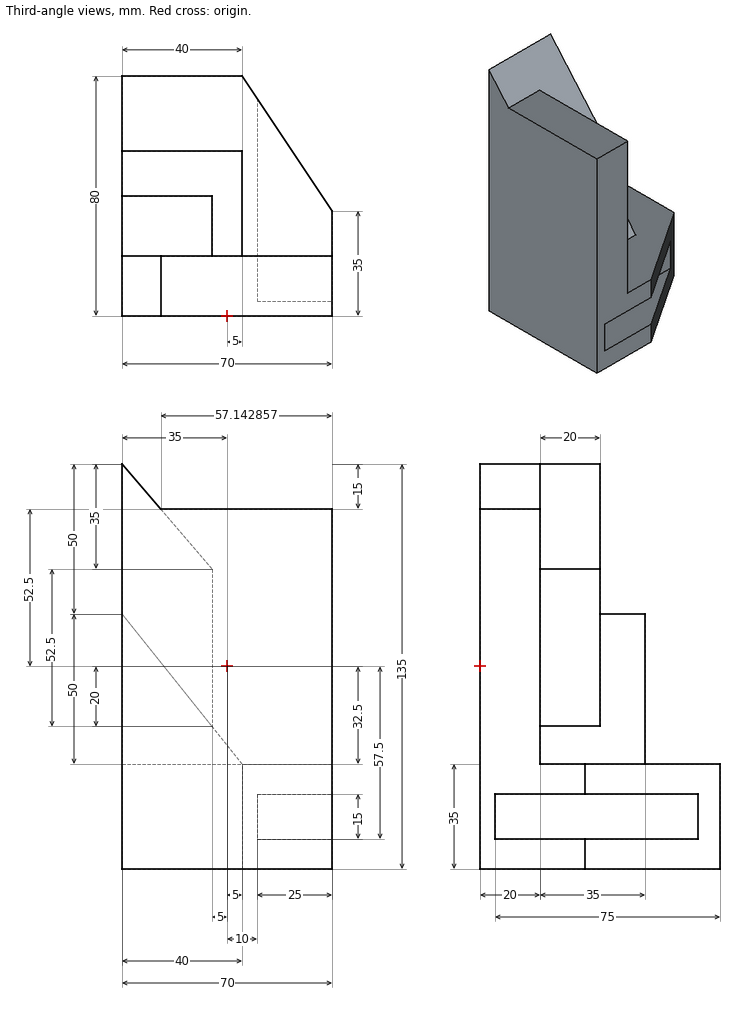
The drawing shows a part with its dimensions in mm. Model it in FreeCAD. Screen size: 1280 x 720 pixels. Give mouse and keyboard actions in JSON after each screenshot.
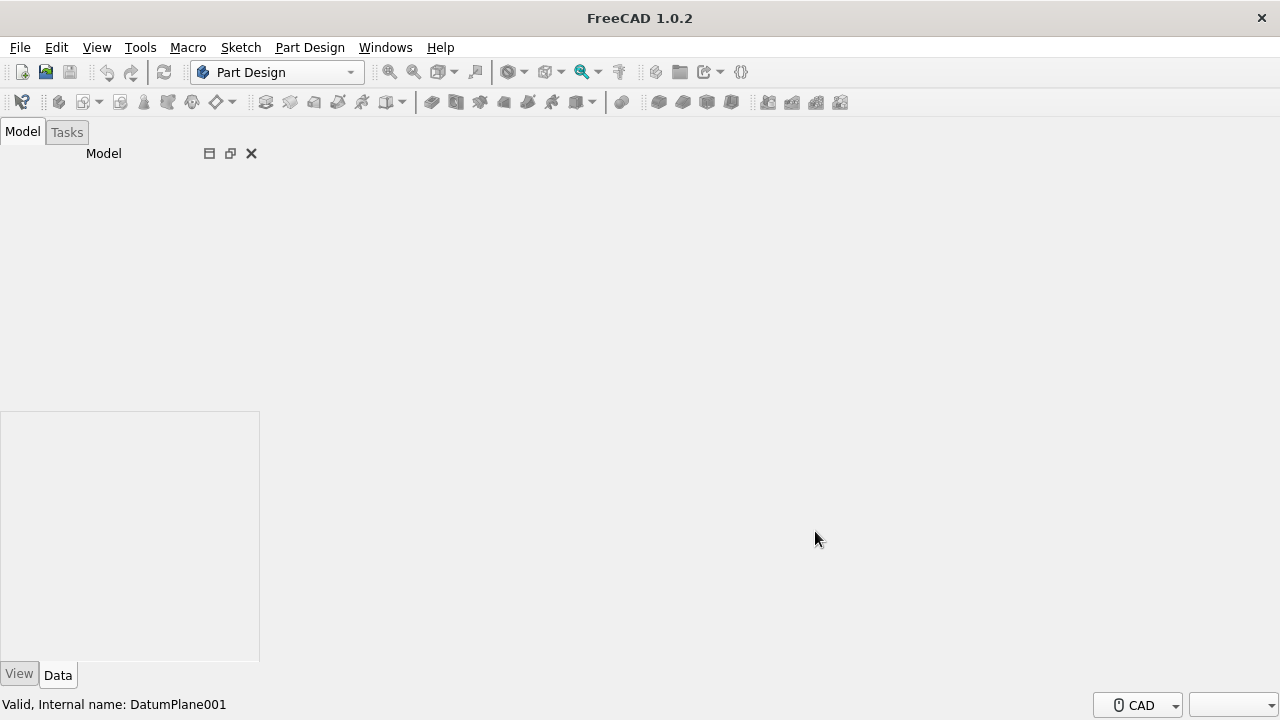
{"action": "left_click", "coordinate": [22, 72]}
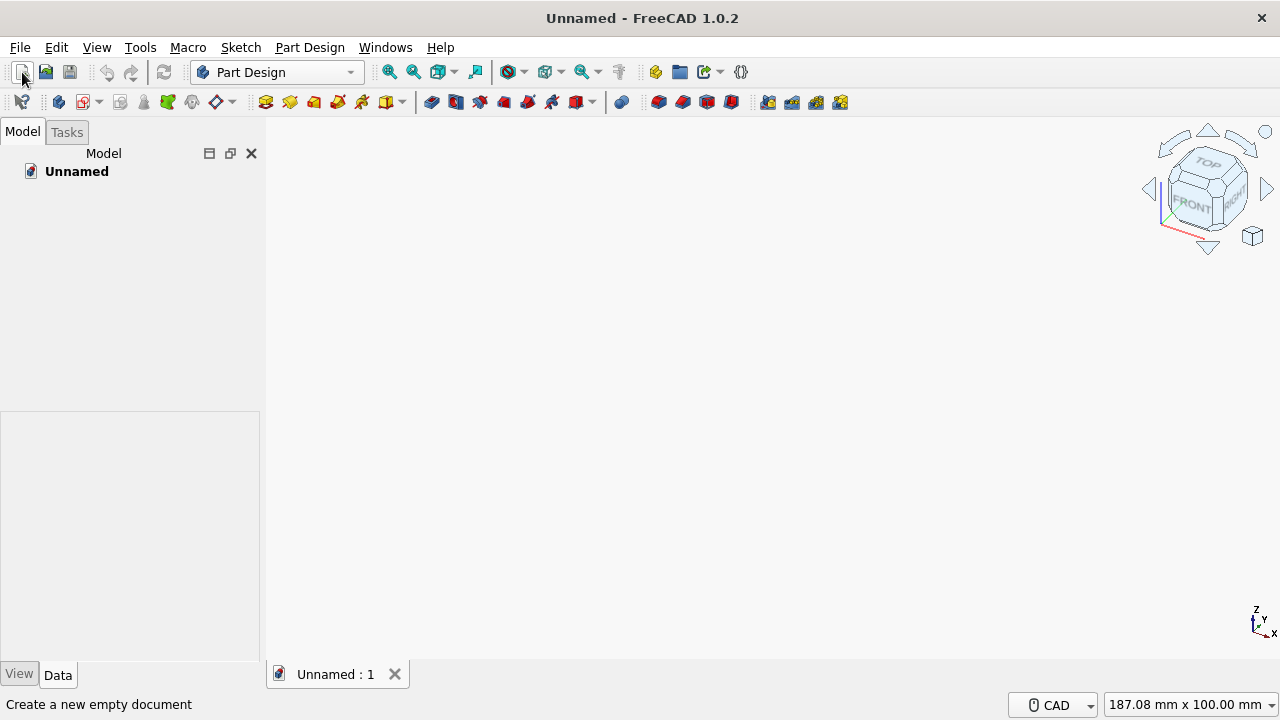
{"action": "left_click", "coordinate": [84, 102]}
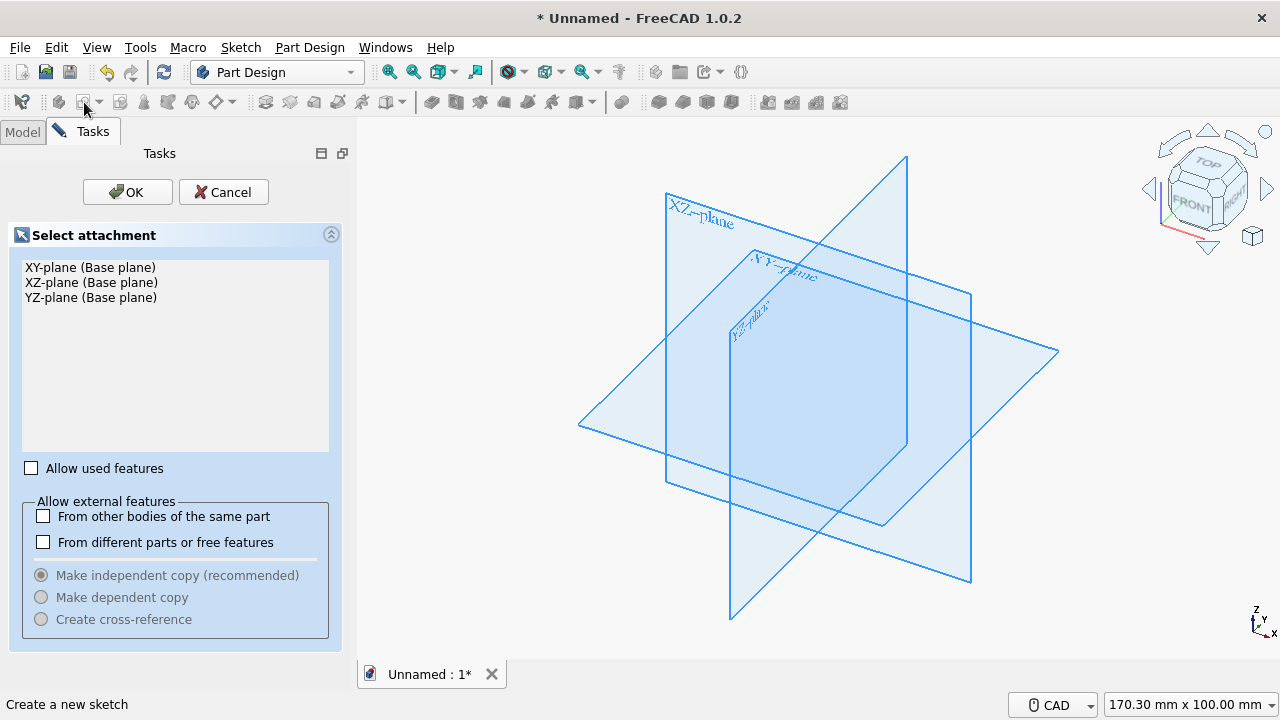
{"action": "left_click", "coordinate": [82, 282]}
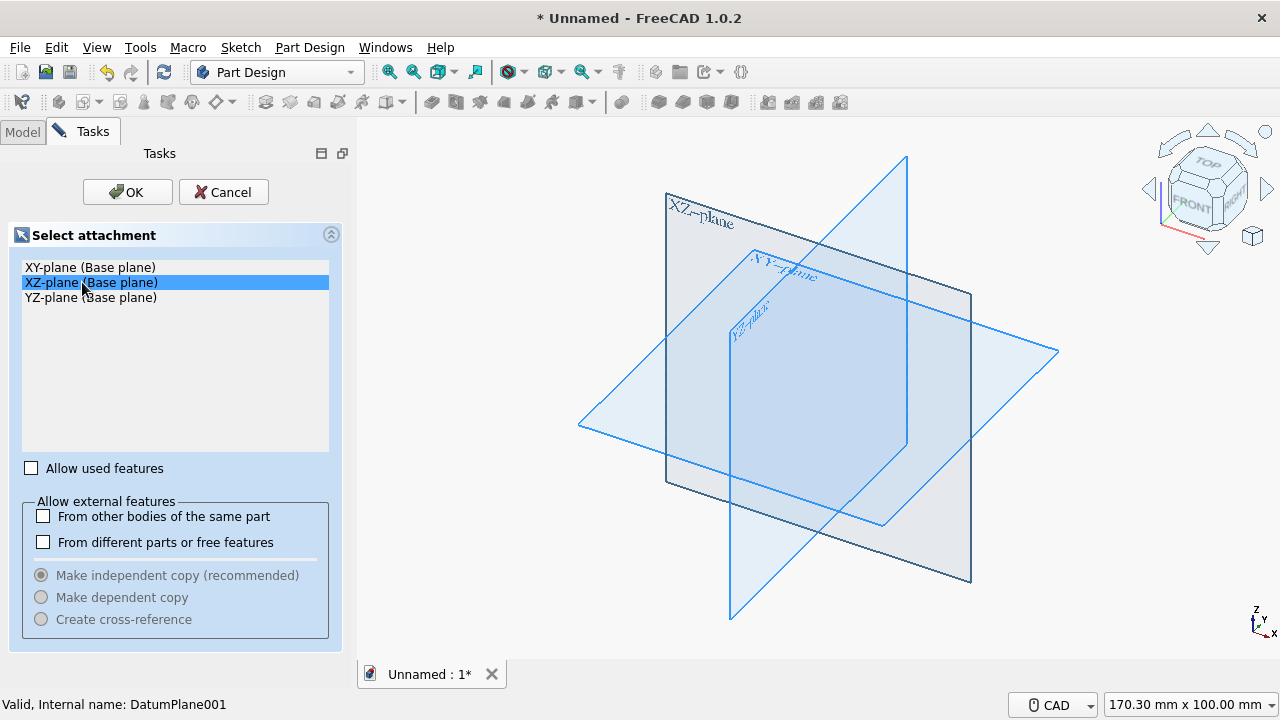
{"action": "left_click", "coordinate": [128, 192]}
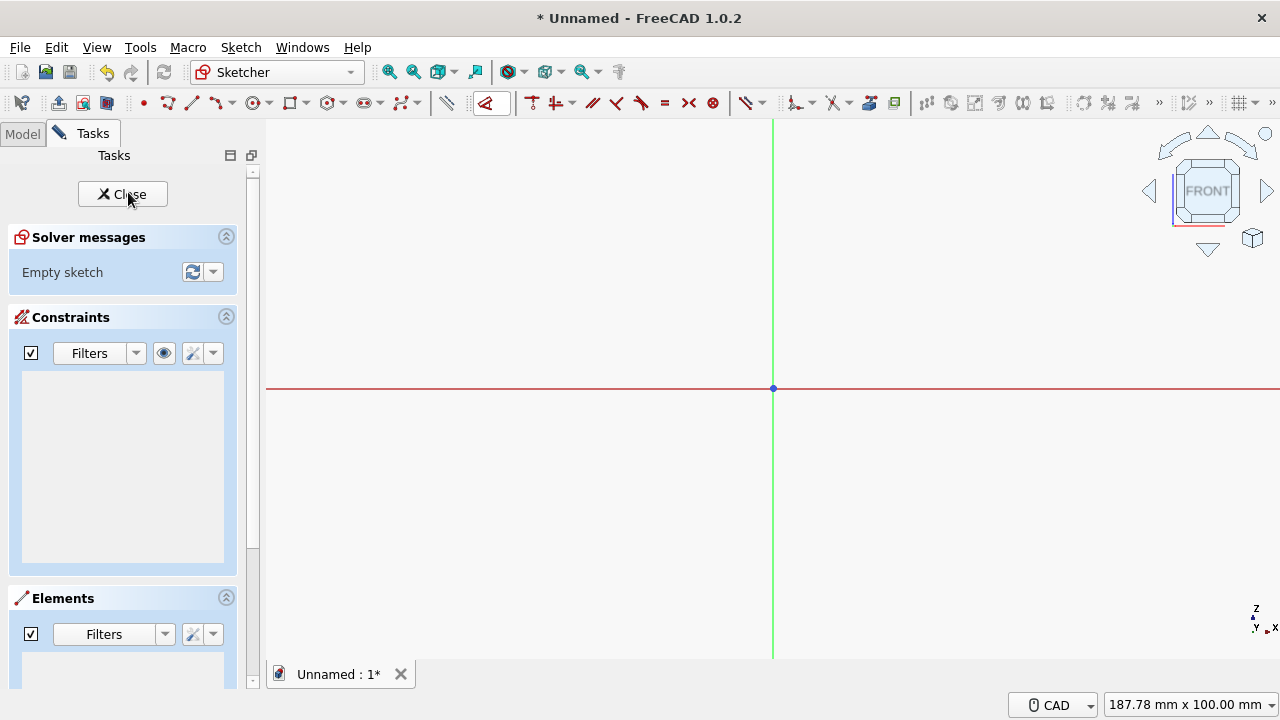
{"action": "scroll", "coordinate": [649, 389], "scroll_direction": "down", "scroll_amount": 4}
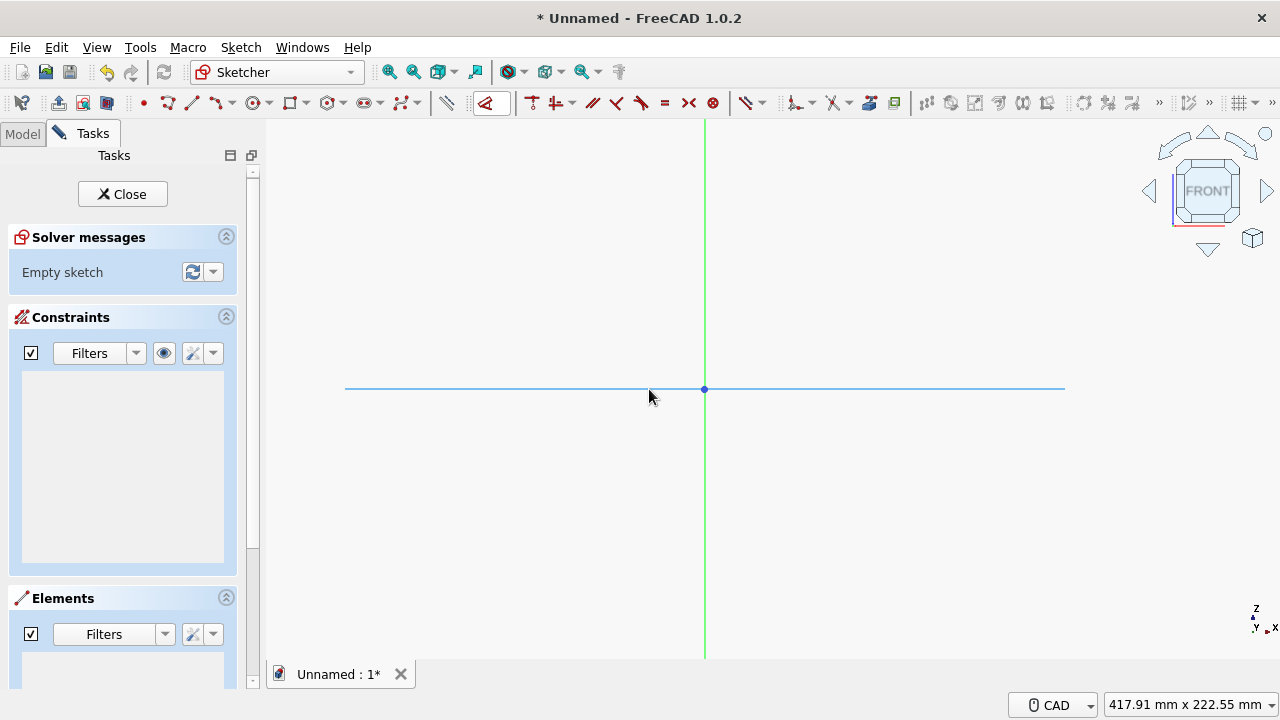
{"action": "key", "text": "g v"}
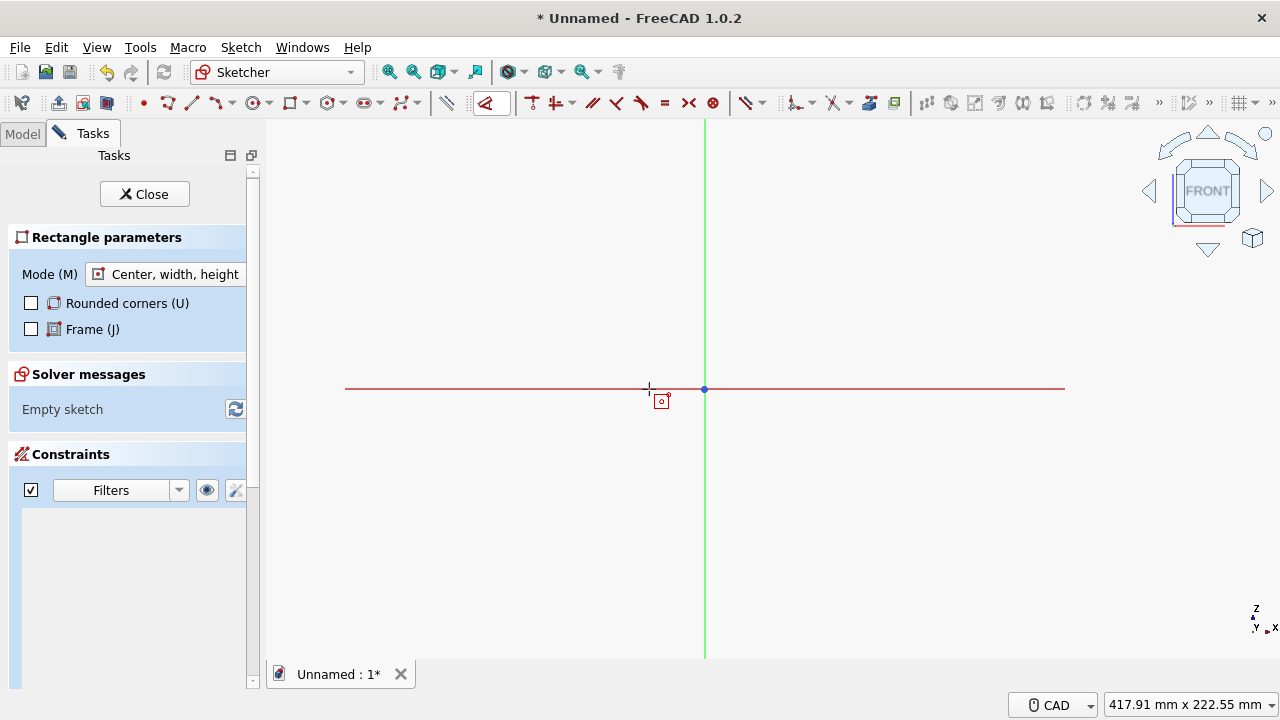
{"action": "left_click", "coordinate": [705, 389]}
{"action": "left_click", "coordinate": [790, 225]}
{"action": "key", "text": "Escape"}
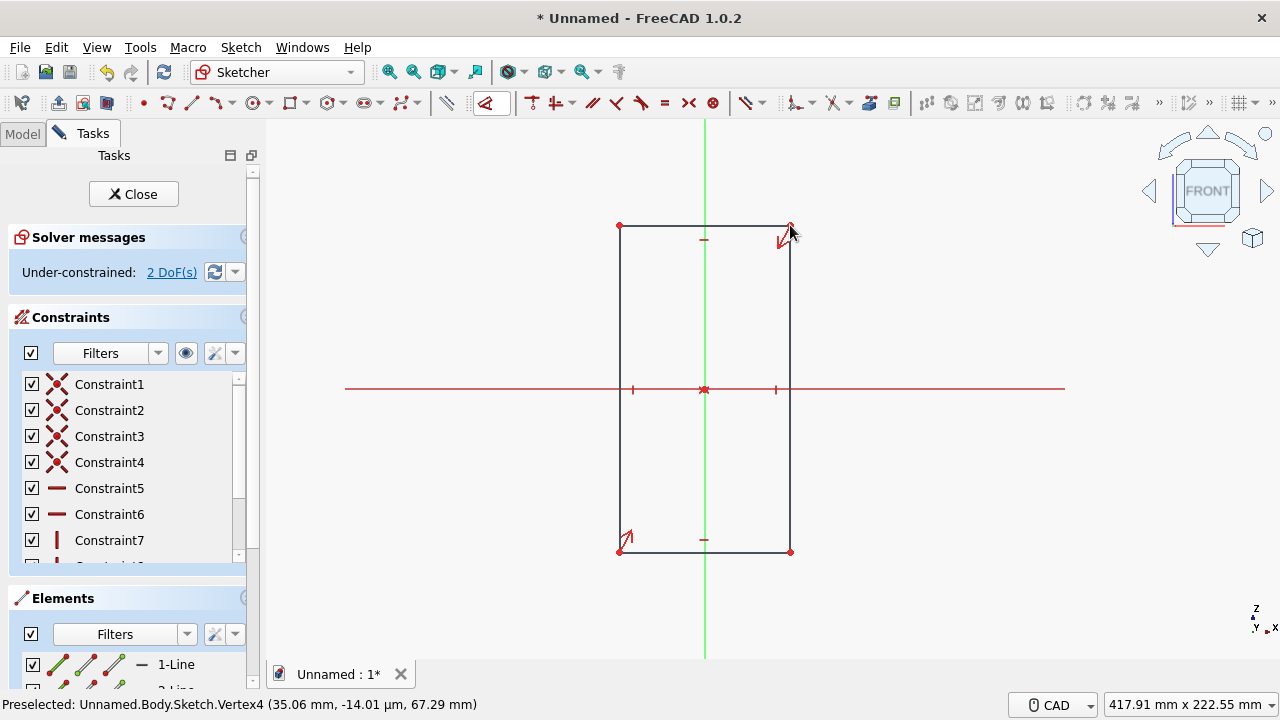
{"action": "left_click", "coordinate": [671, 553]}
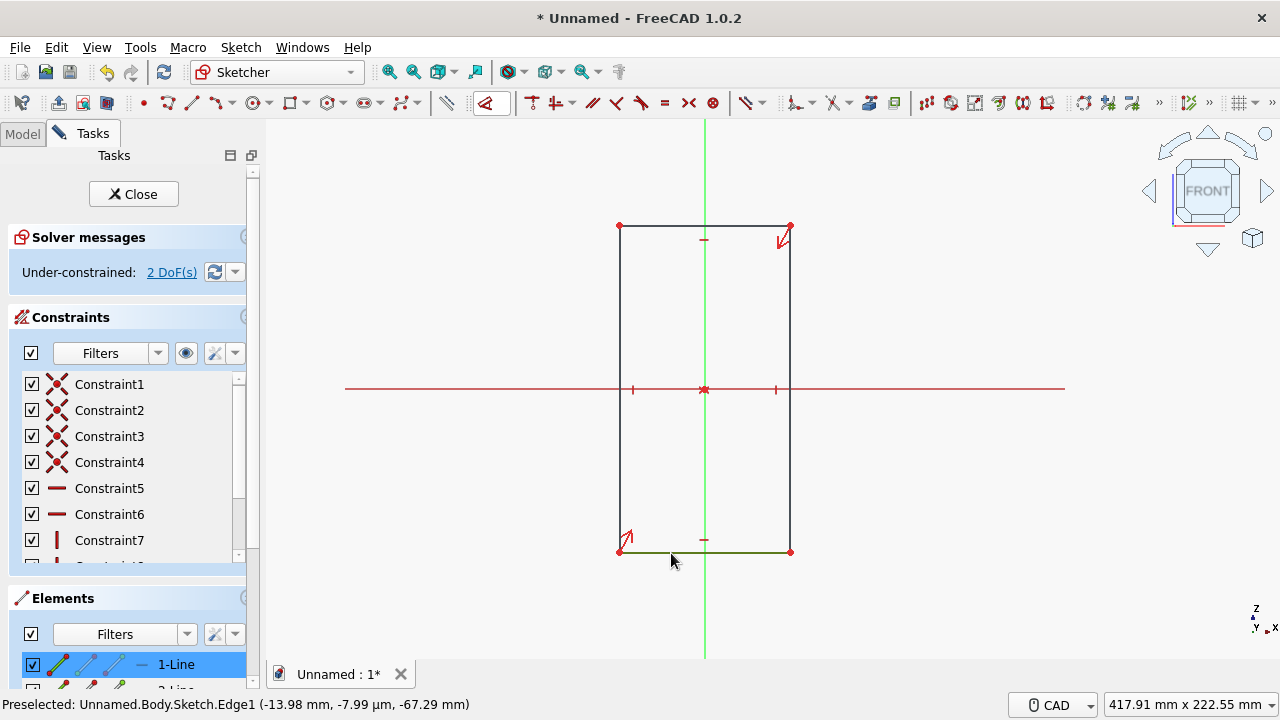
{"action": "key", "text": "l"}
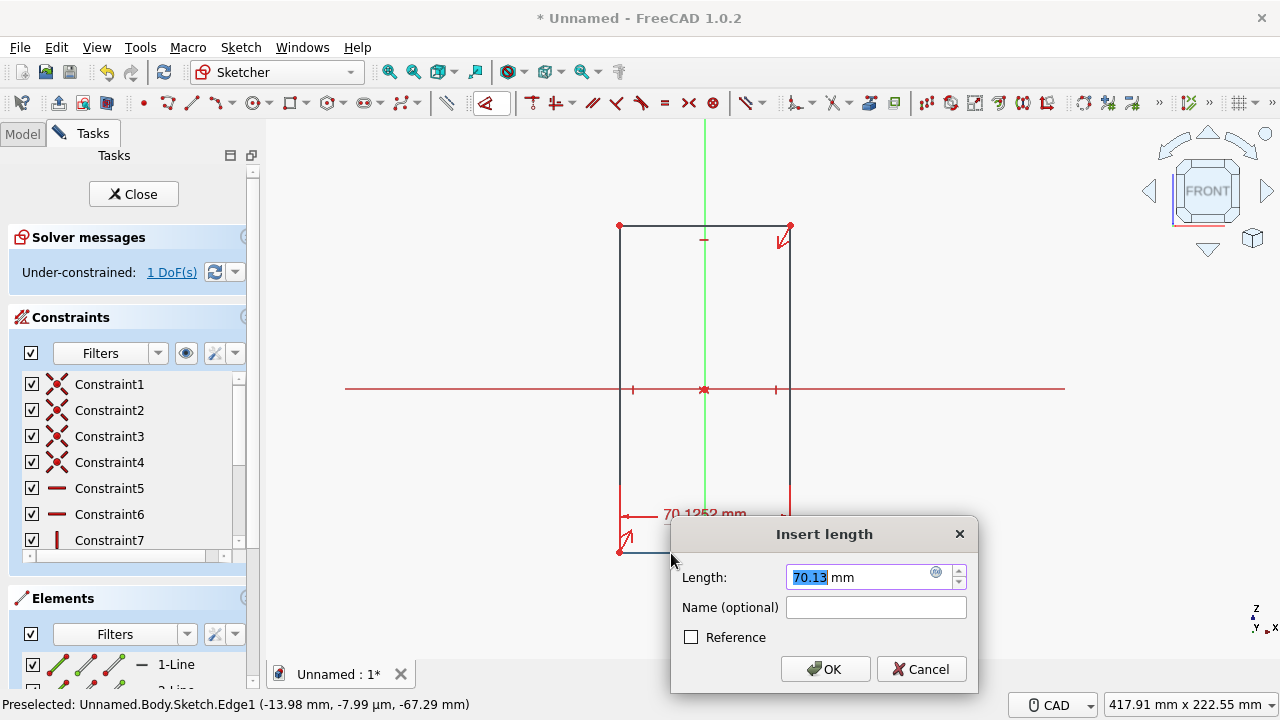
{"action": "type", "text": "70"}
{"action": "key", "text": "Return"}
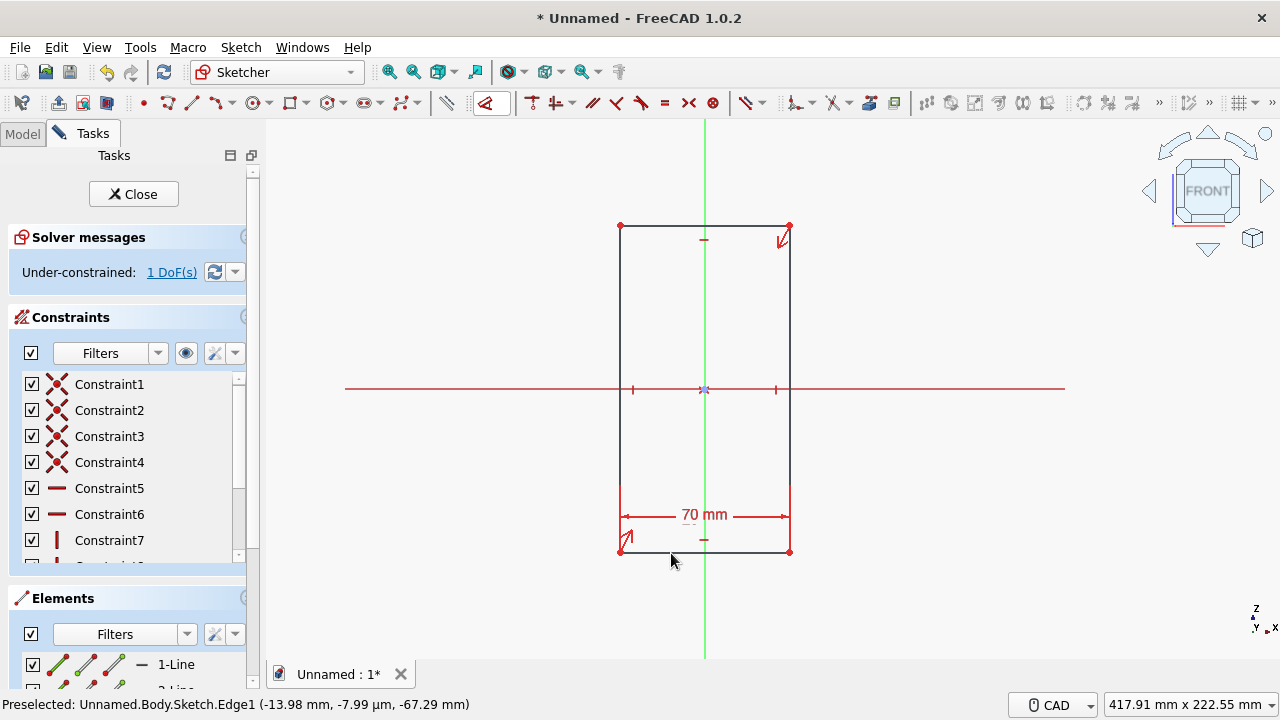
{"action": "left_click", "coordinate": [790, 455]}